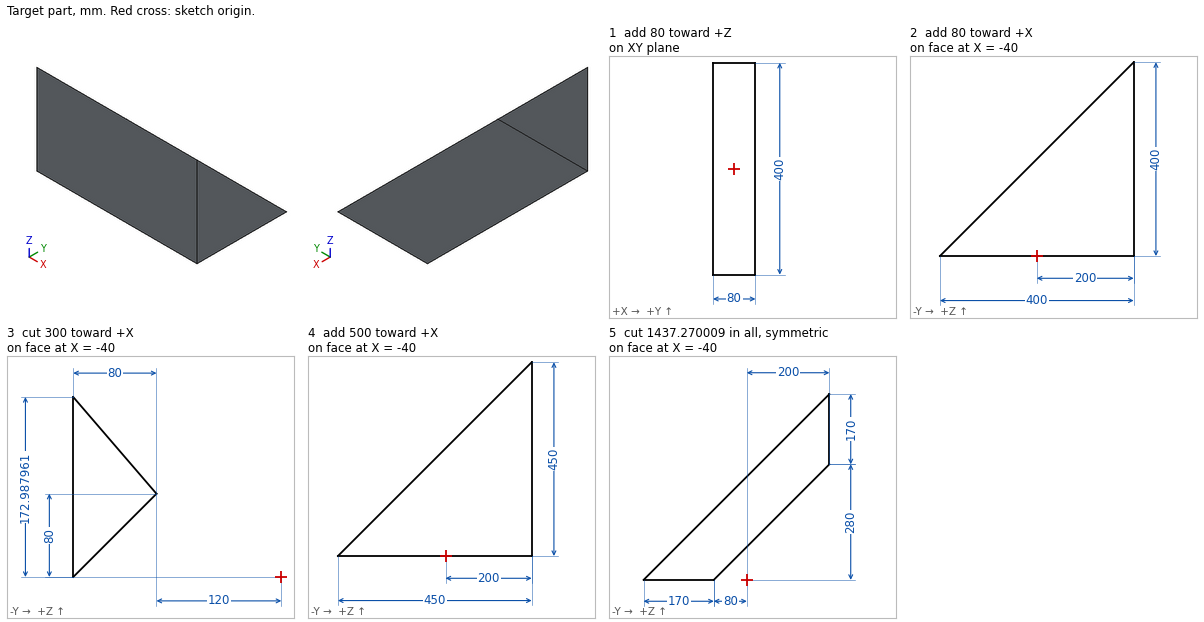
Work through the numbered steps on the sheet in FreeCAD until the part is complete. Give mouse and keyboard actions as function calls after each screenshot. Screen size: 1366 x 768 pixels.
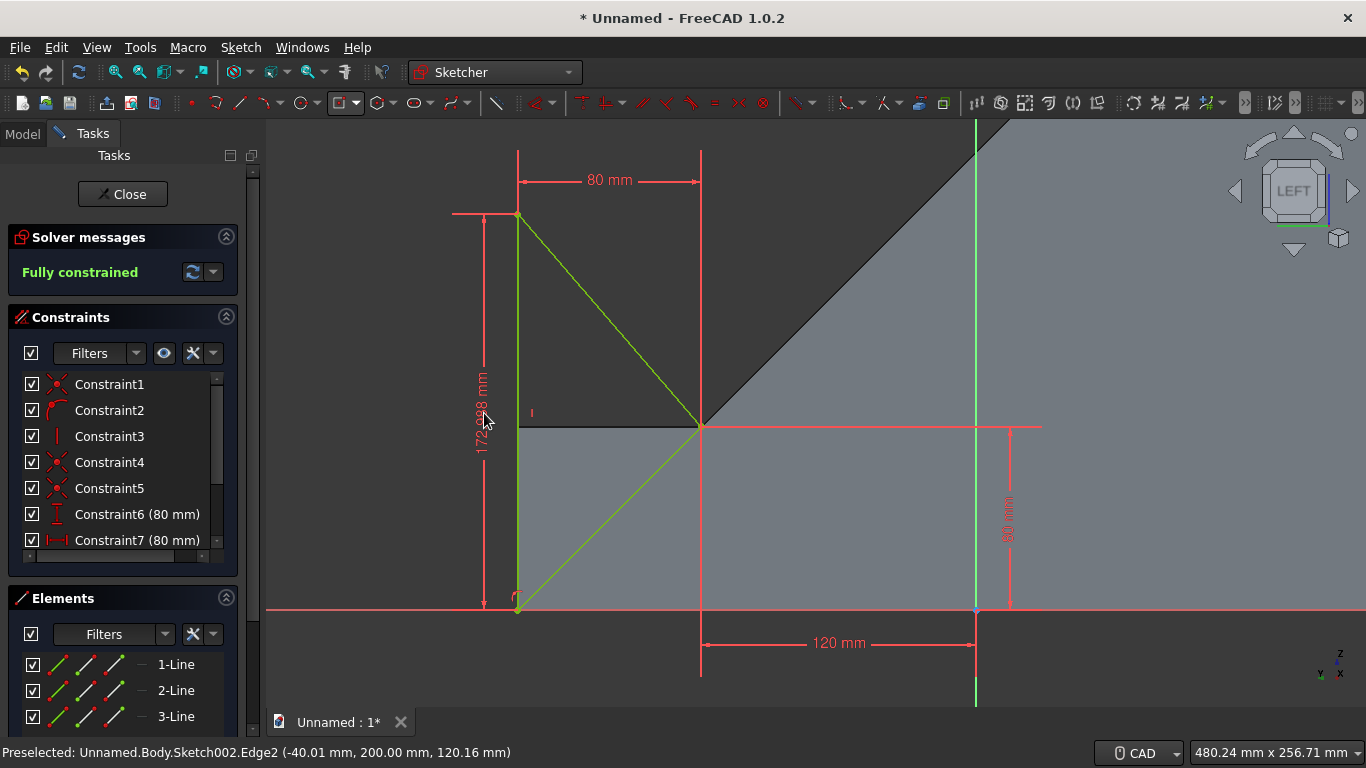
click(123, 194)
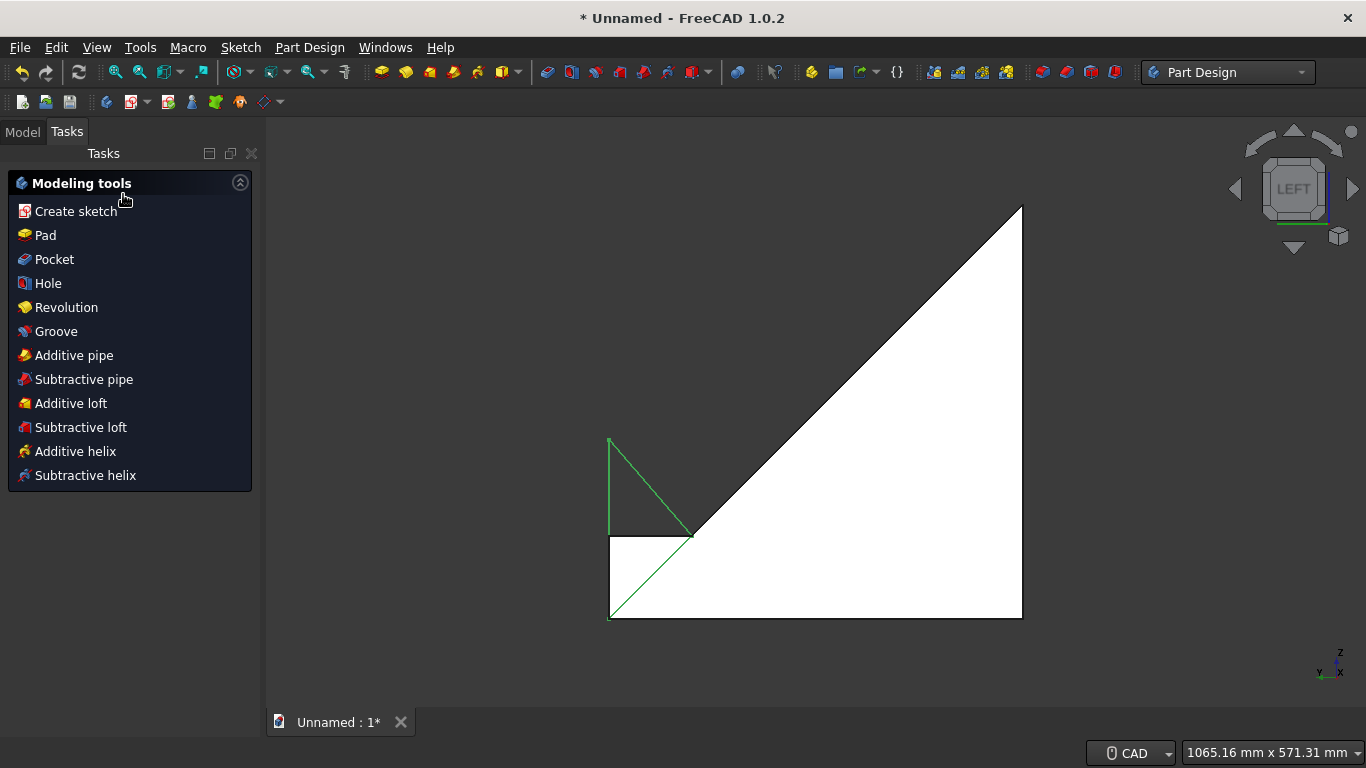
click(548, 72)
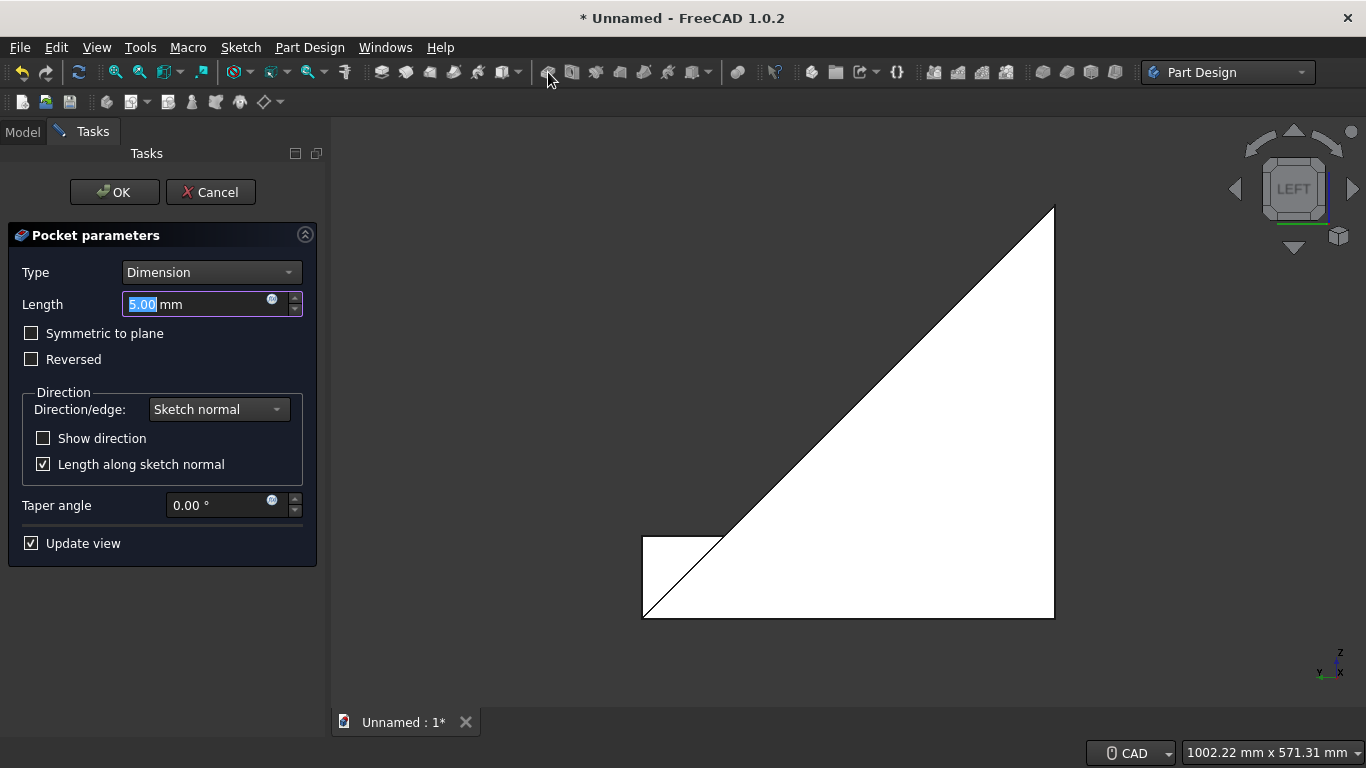
text(300)
key(Tab)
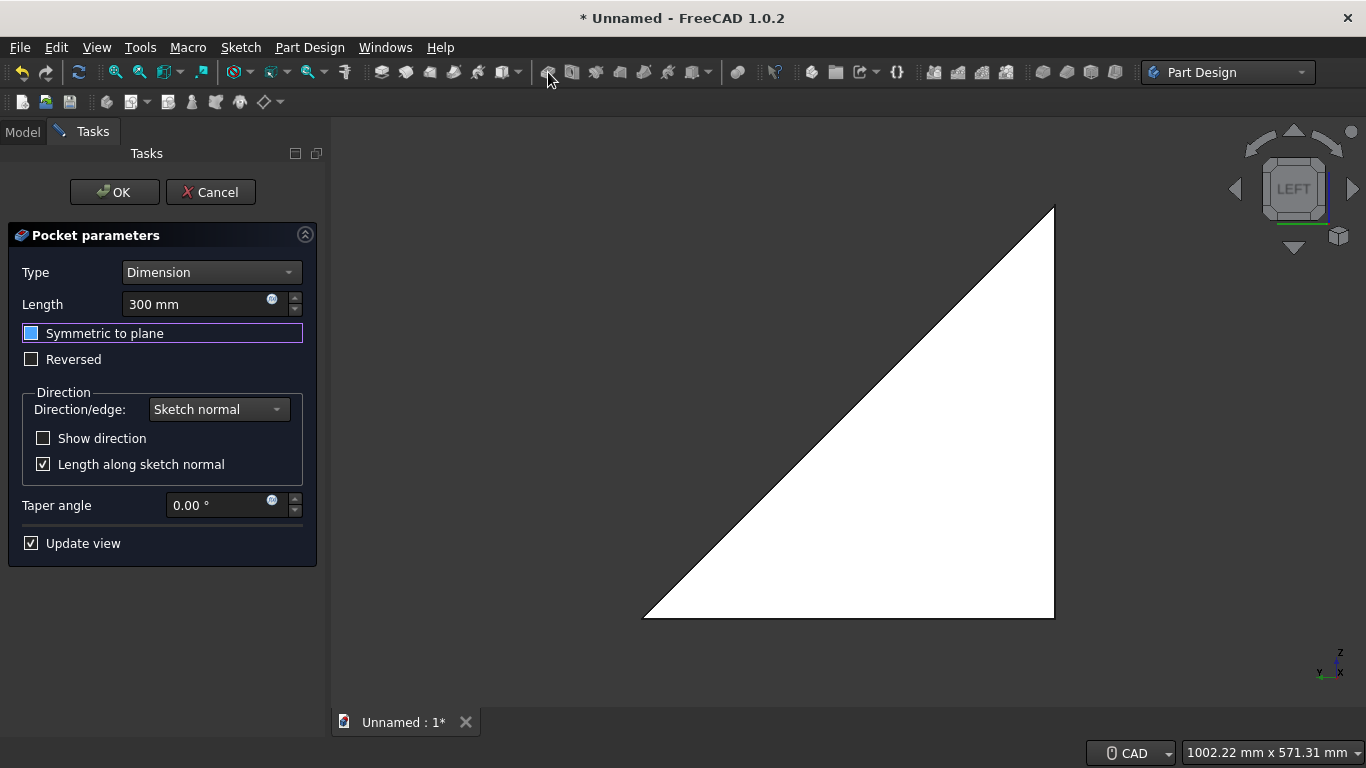
click(115, 192)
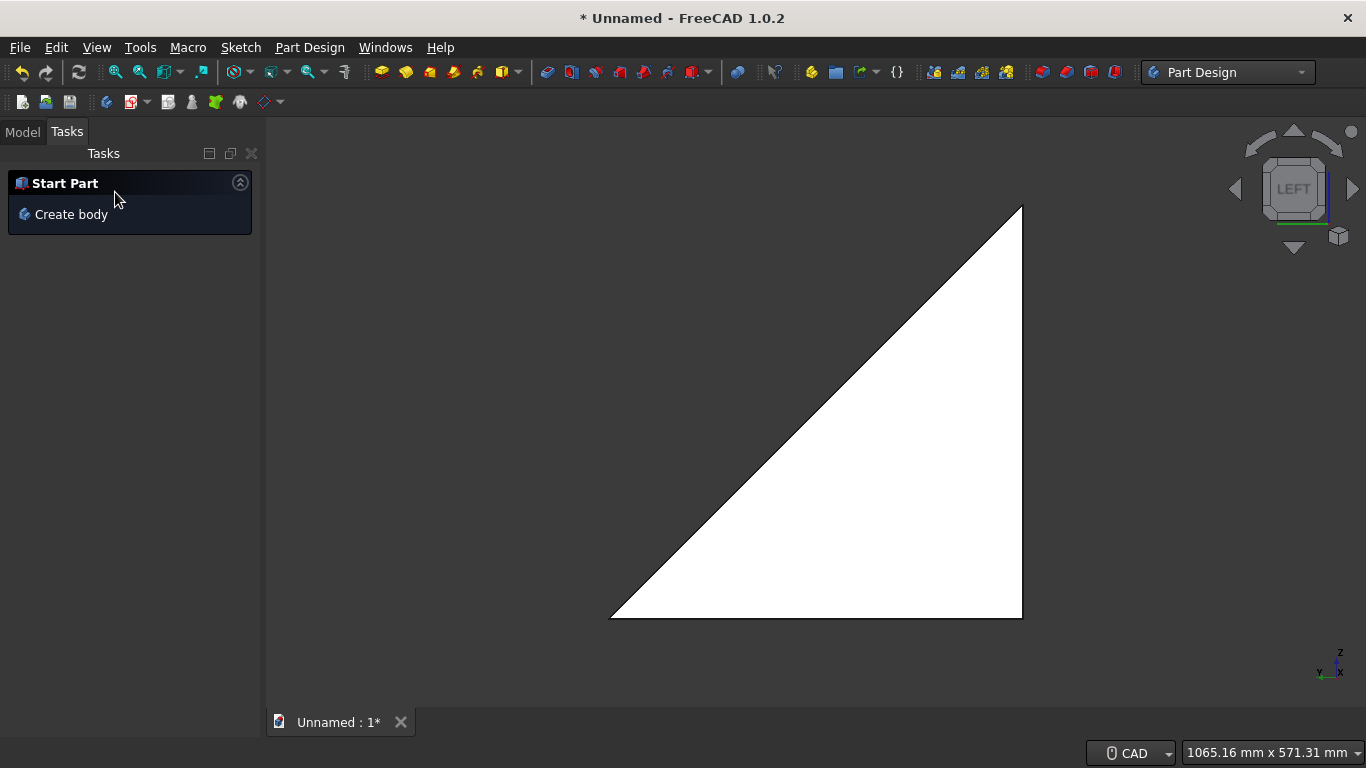
click(934, 470)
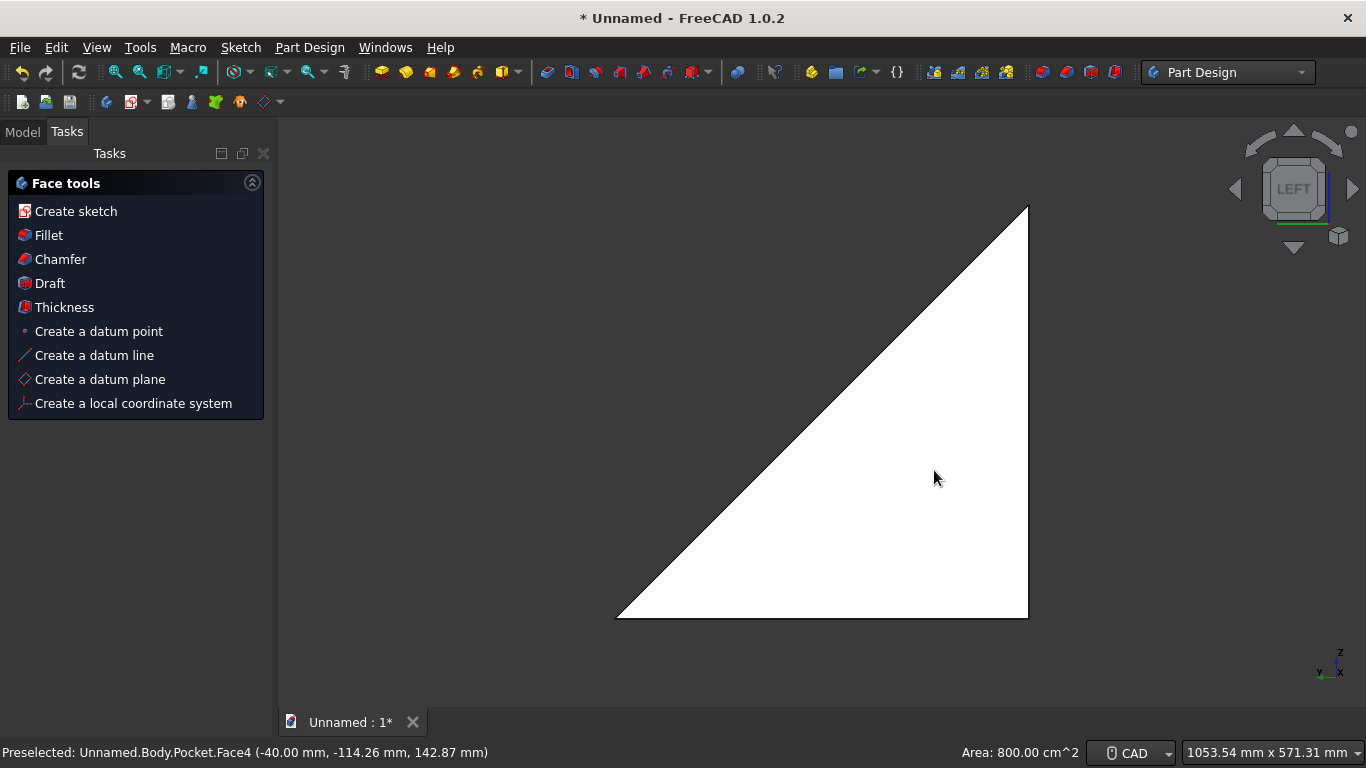
click(132, 102)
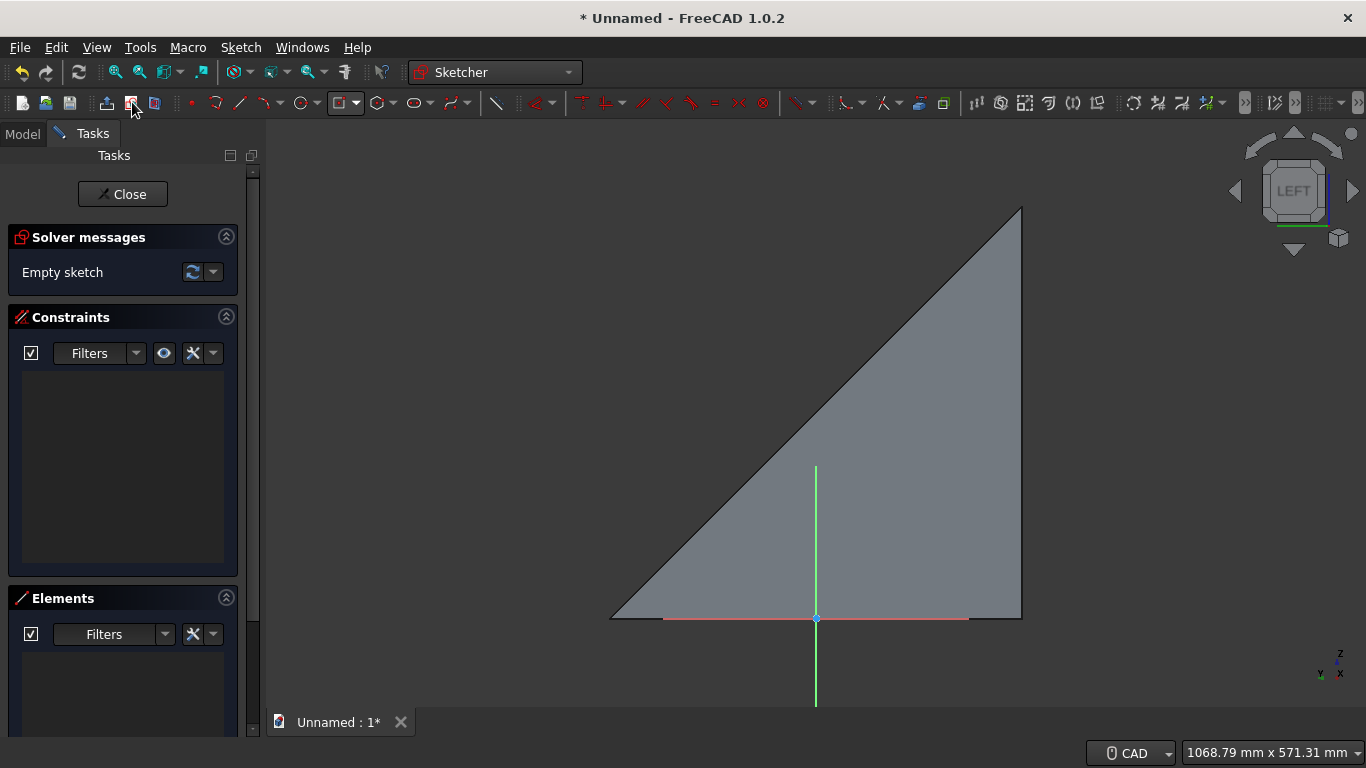
scroll(554, 529, down, 1)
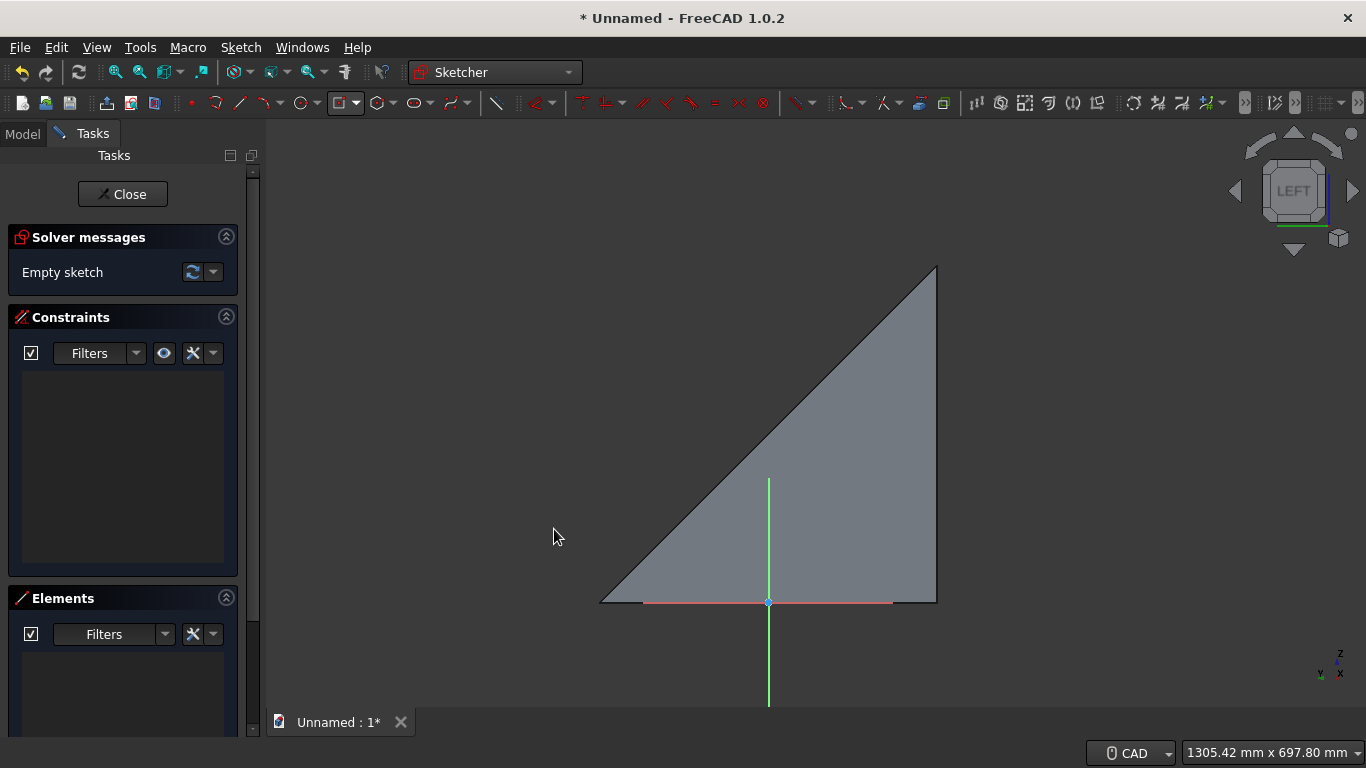
click(216, 104)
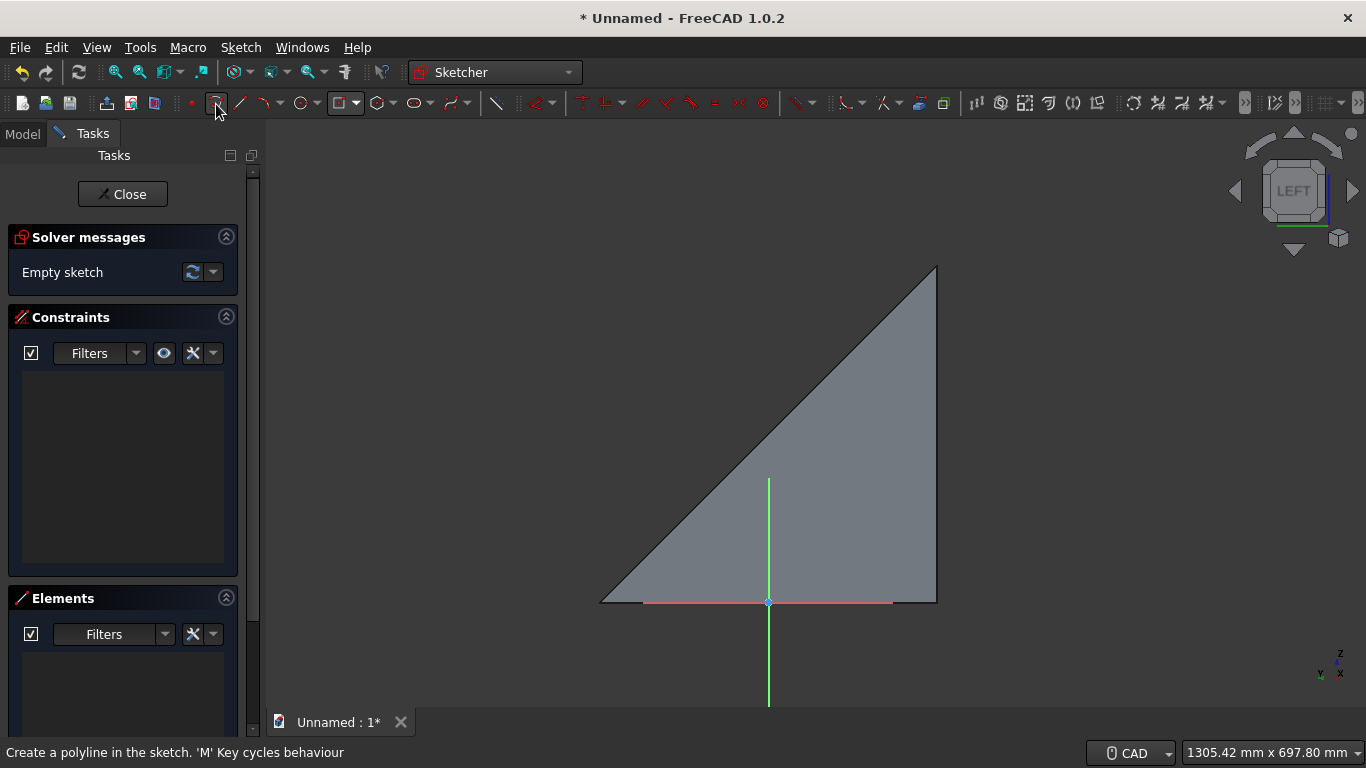
click(937, 603)
click(937, 223)
click(558, 594)
click(937, 604)
key(Escape)
key(Escape)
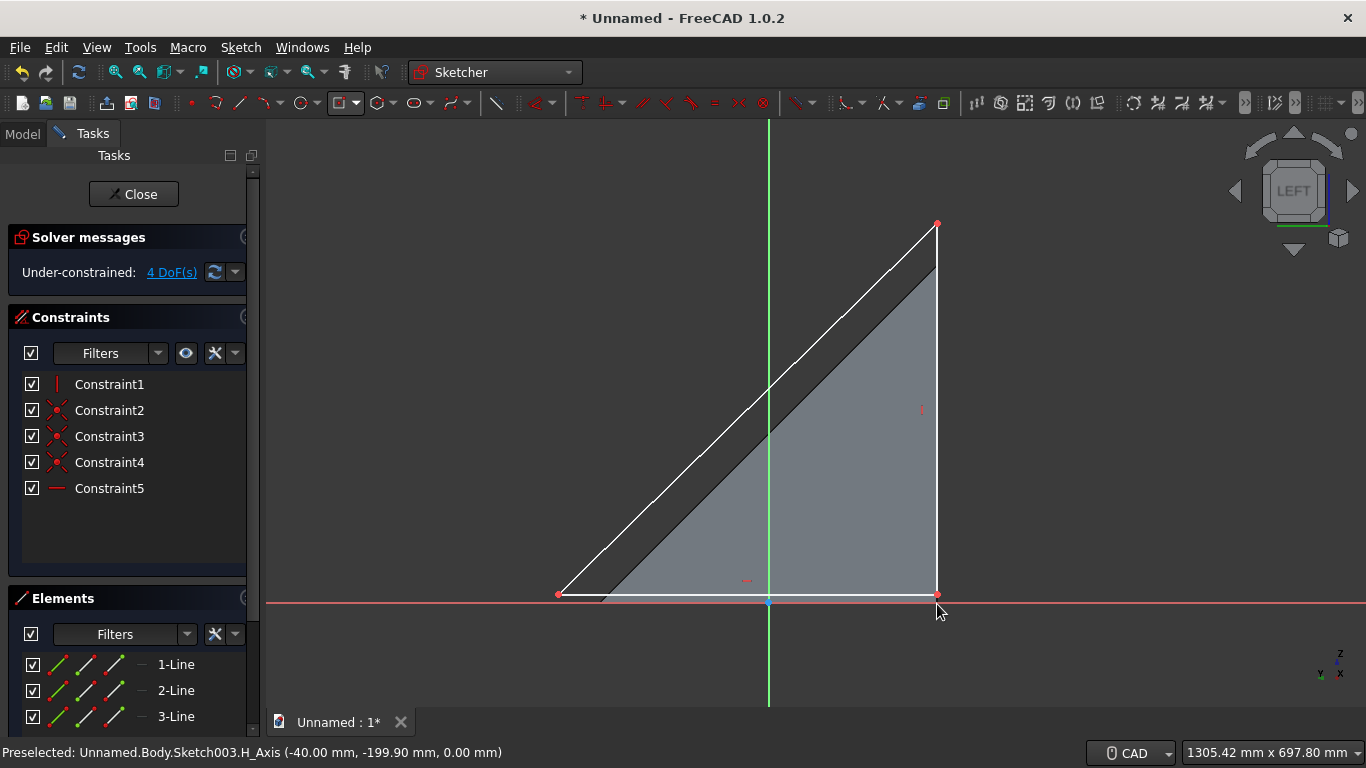
click(937, 595)